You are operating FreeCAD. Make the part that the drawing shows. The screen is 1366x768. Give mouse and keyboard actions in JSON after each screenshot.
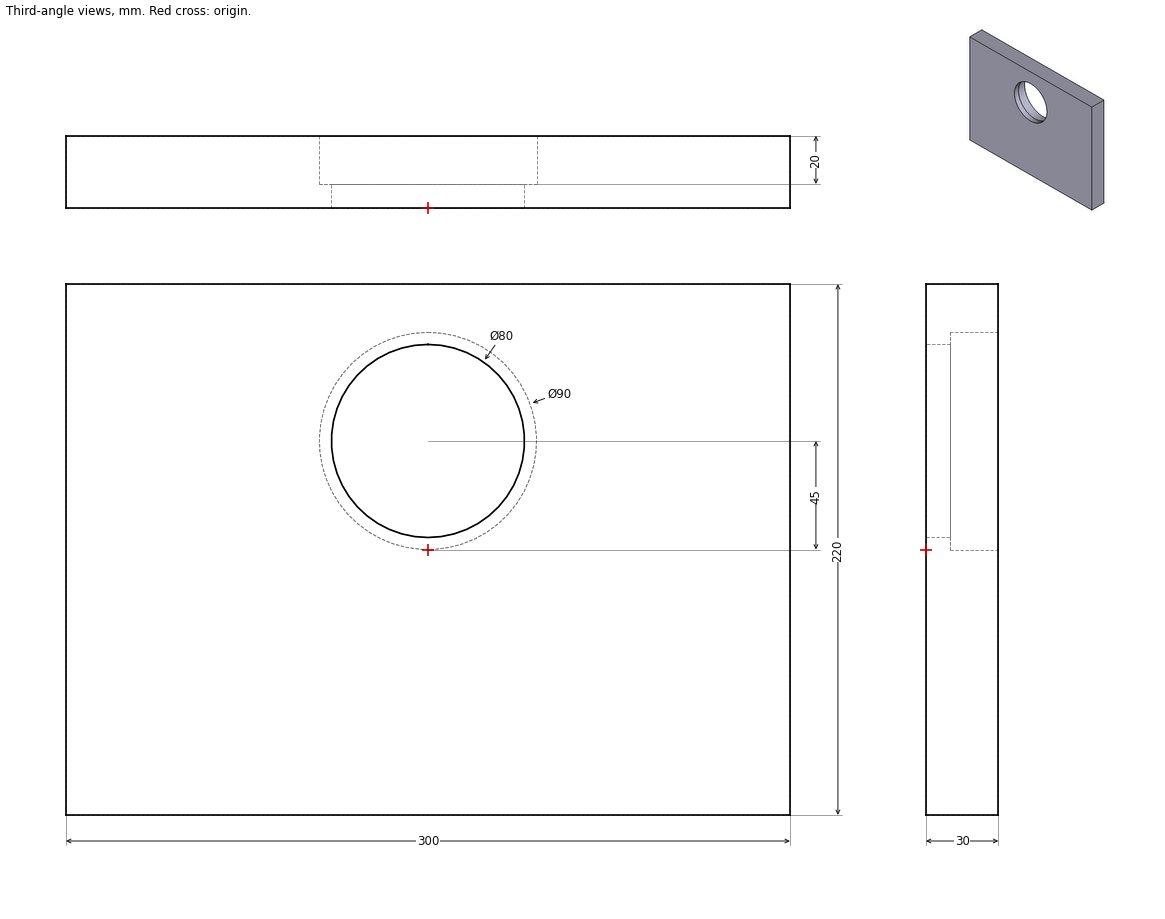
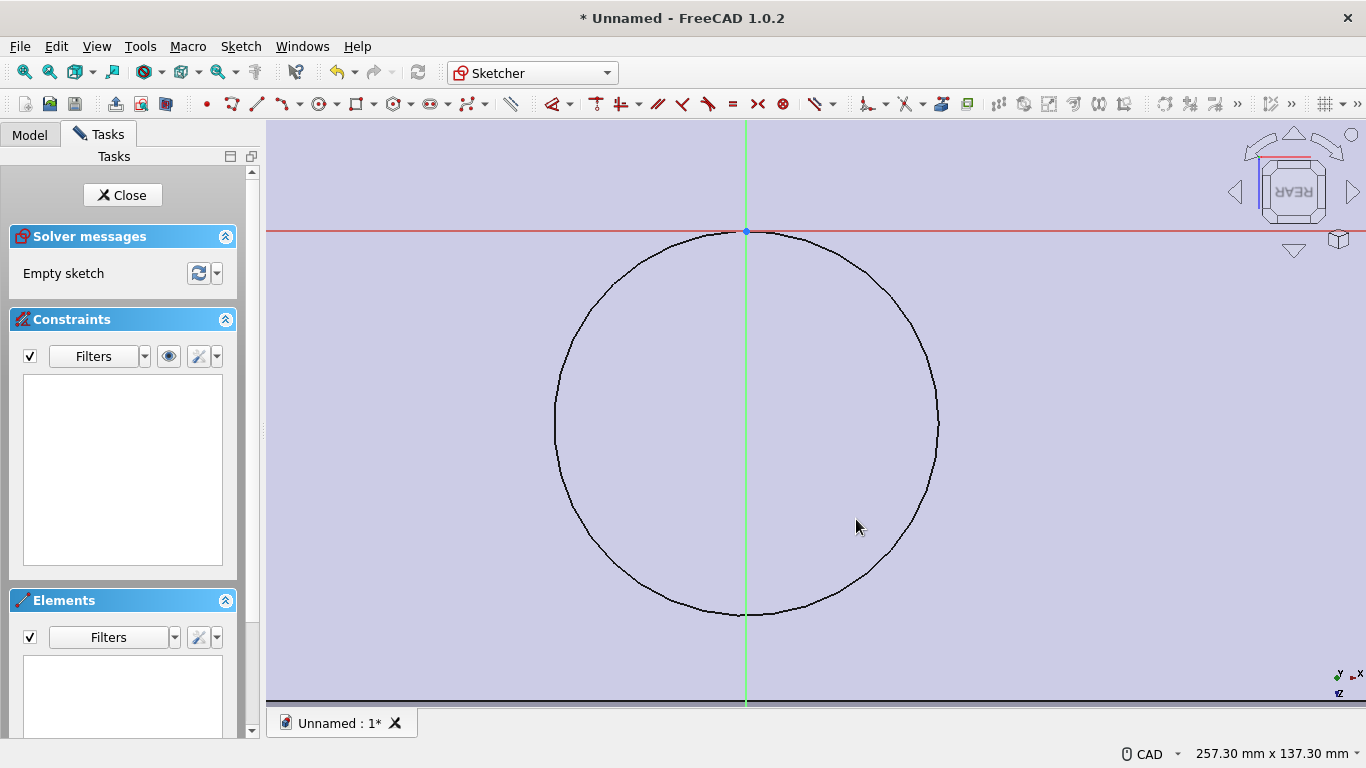
{"action": "left_click", "coordinate": [318, 104]}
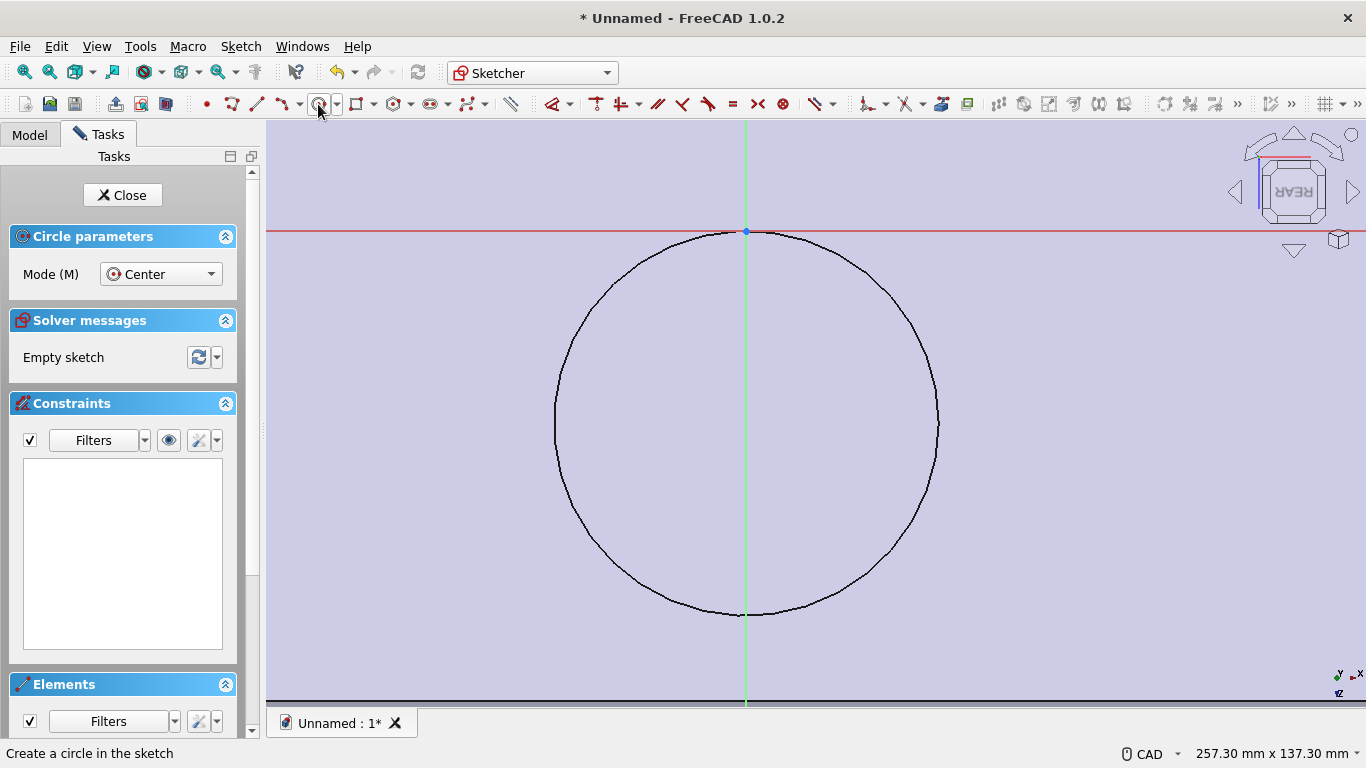
{"action": "left_click", "coordinate": [746, 423]}
{"action": "left_click", "coordinate": [867, 303]}
{"action": "key", "text": "Escape"}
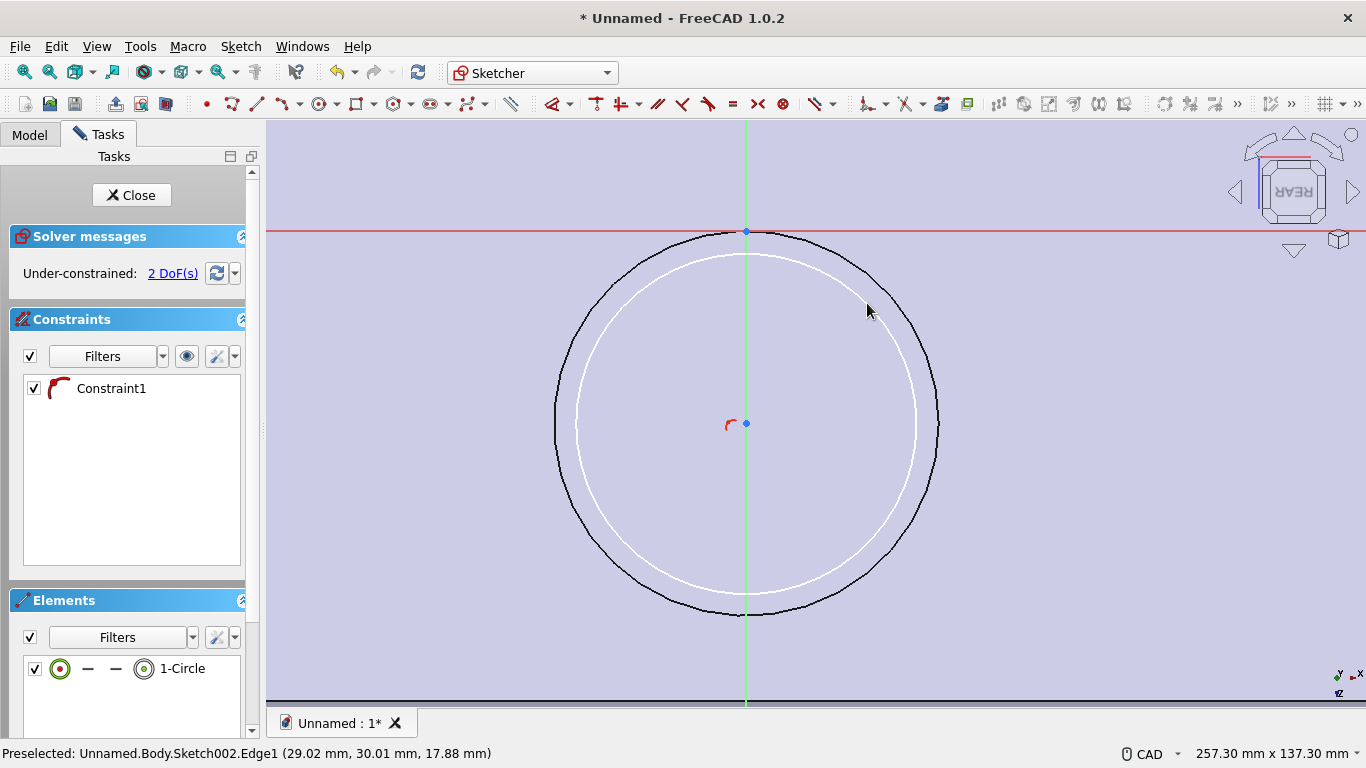
{"action": "left_click", "coordinate": [552, 104]}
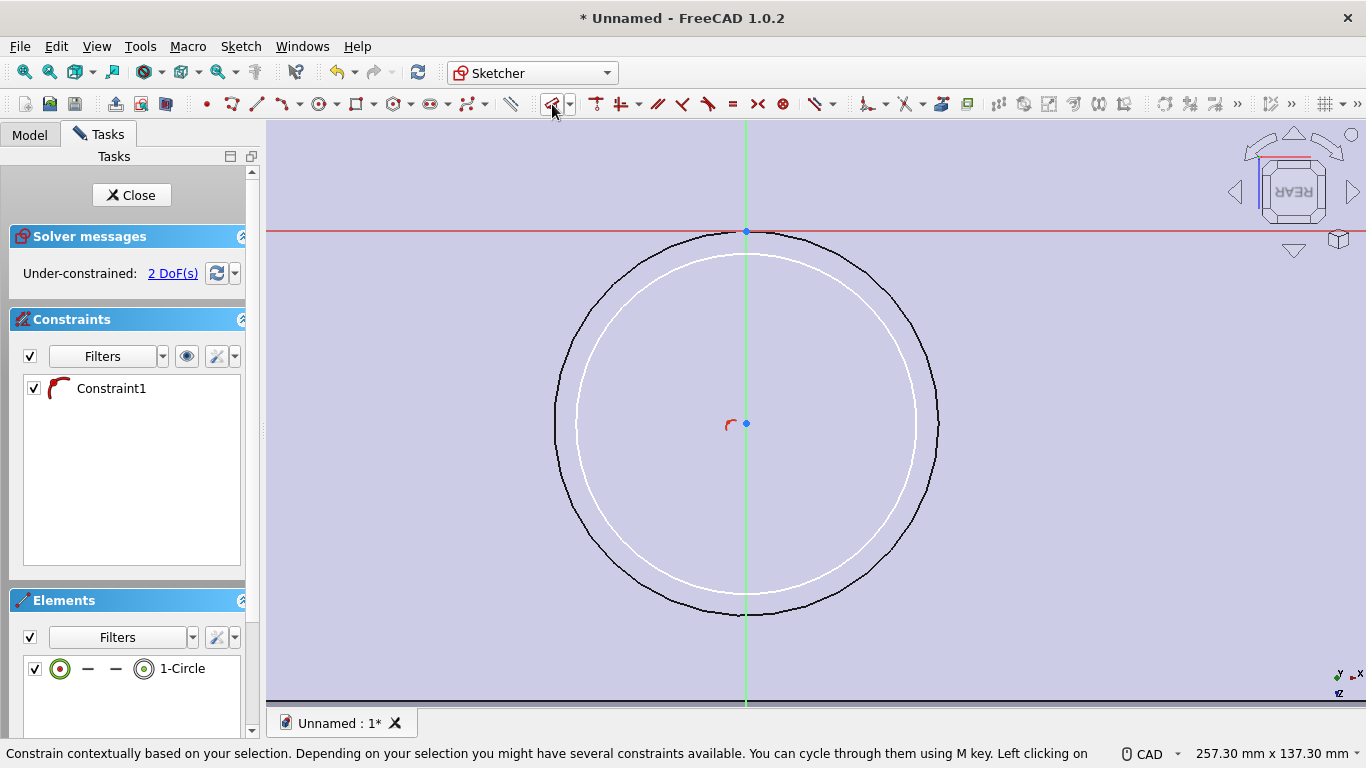
{"action": "left_click", "coordinate": [866, 303]}
{"action": "left_click", "coordinate": [889, 280]}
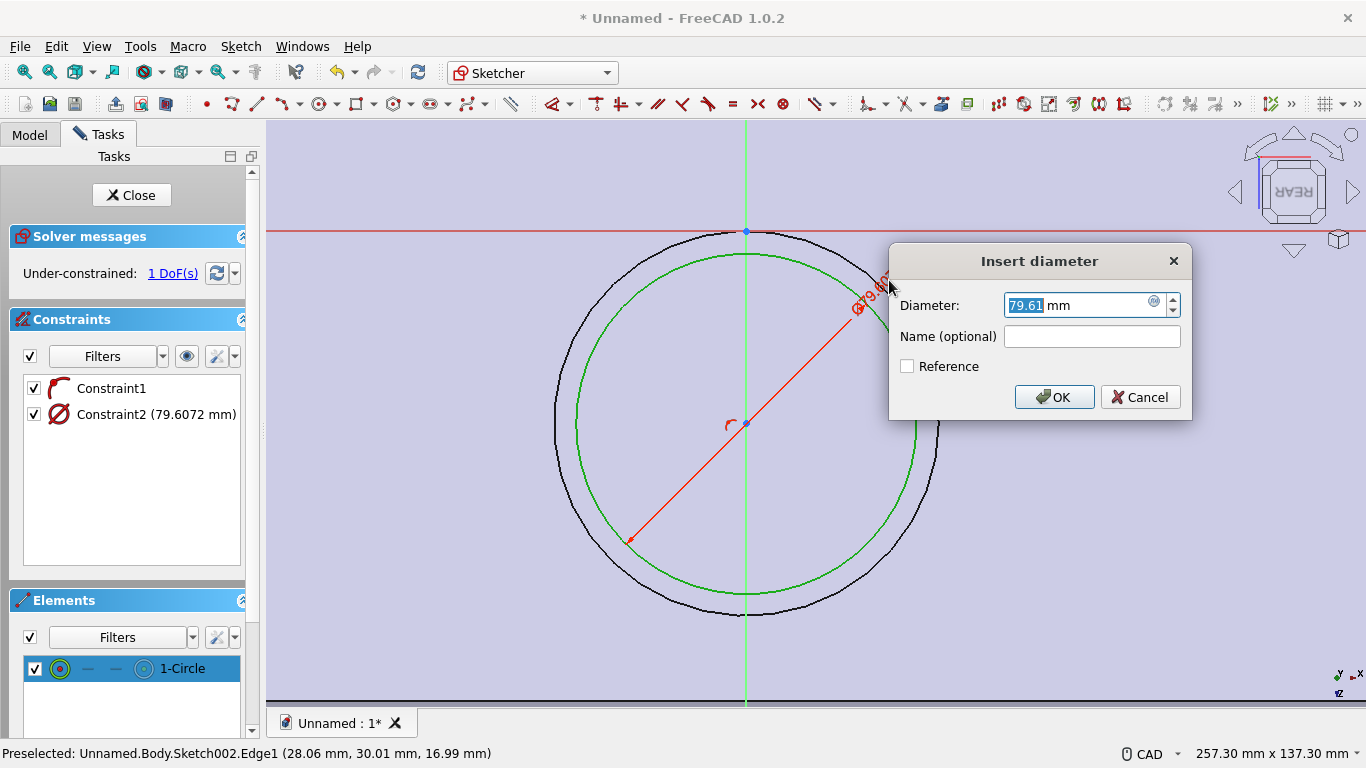
{"action": "type", "text": "80"}
{"action": "key", "text": "Return"}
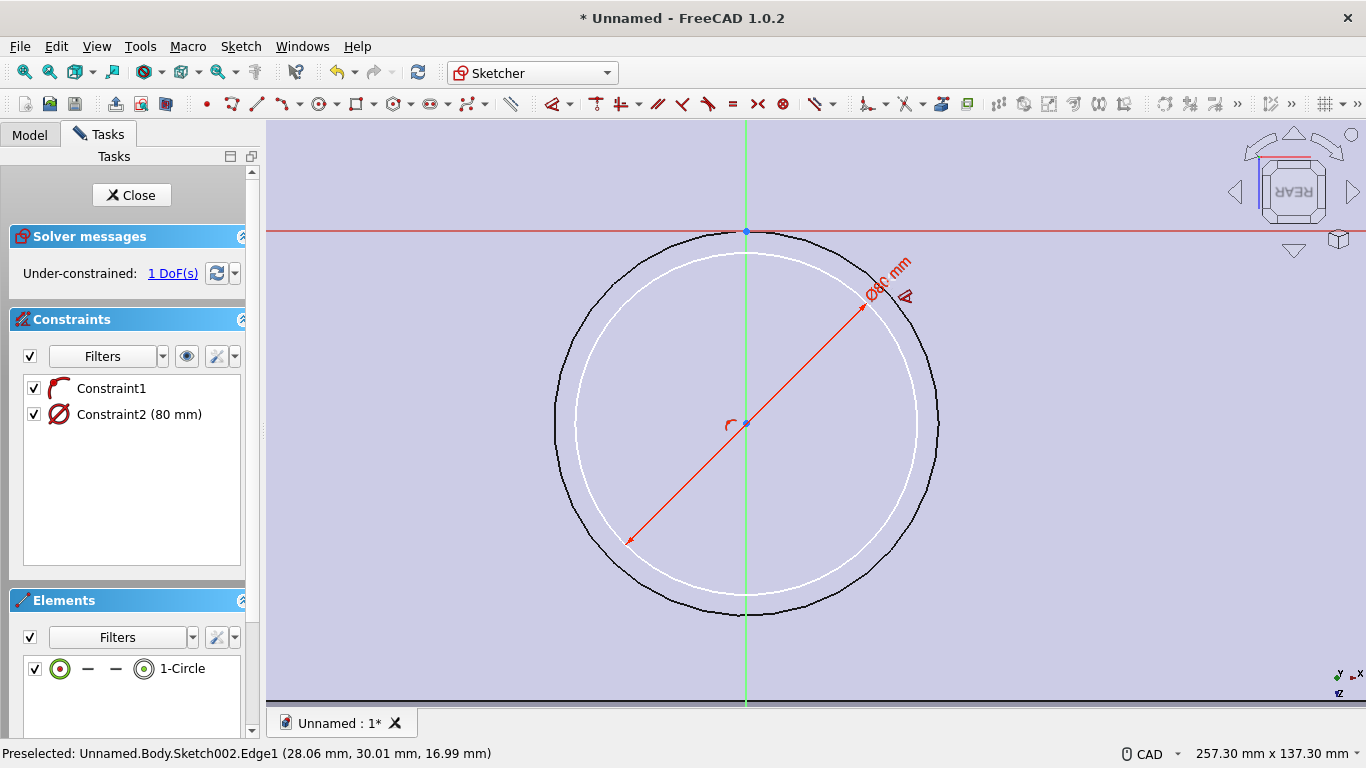
{"action": "left_click", "coordinate": [746, 424]}
{"action": "left_click", "coordinate": [780, 328]}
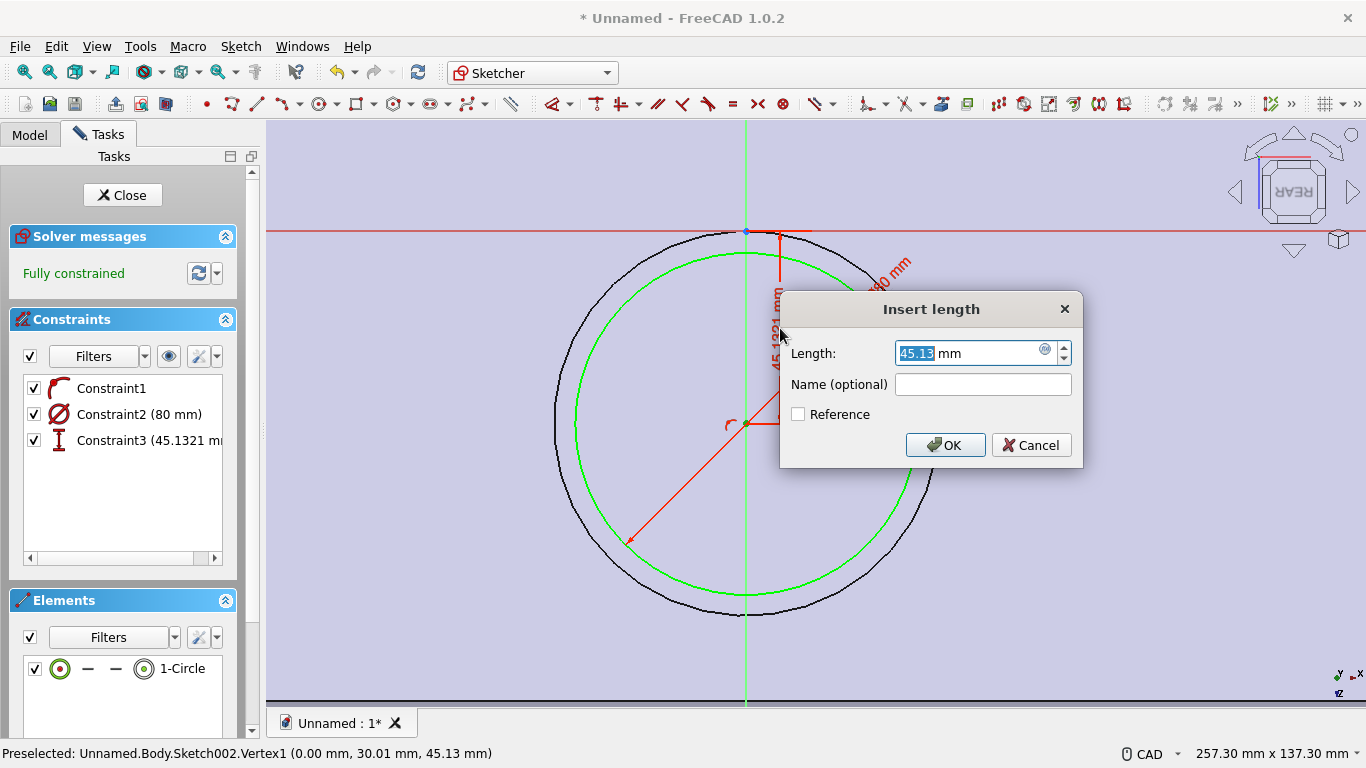
{"action": "type", "text": "45"}
{"action": "key", "text": "Return"}
{"action": "key", "text": "Escape"}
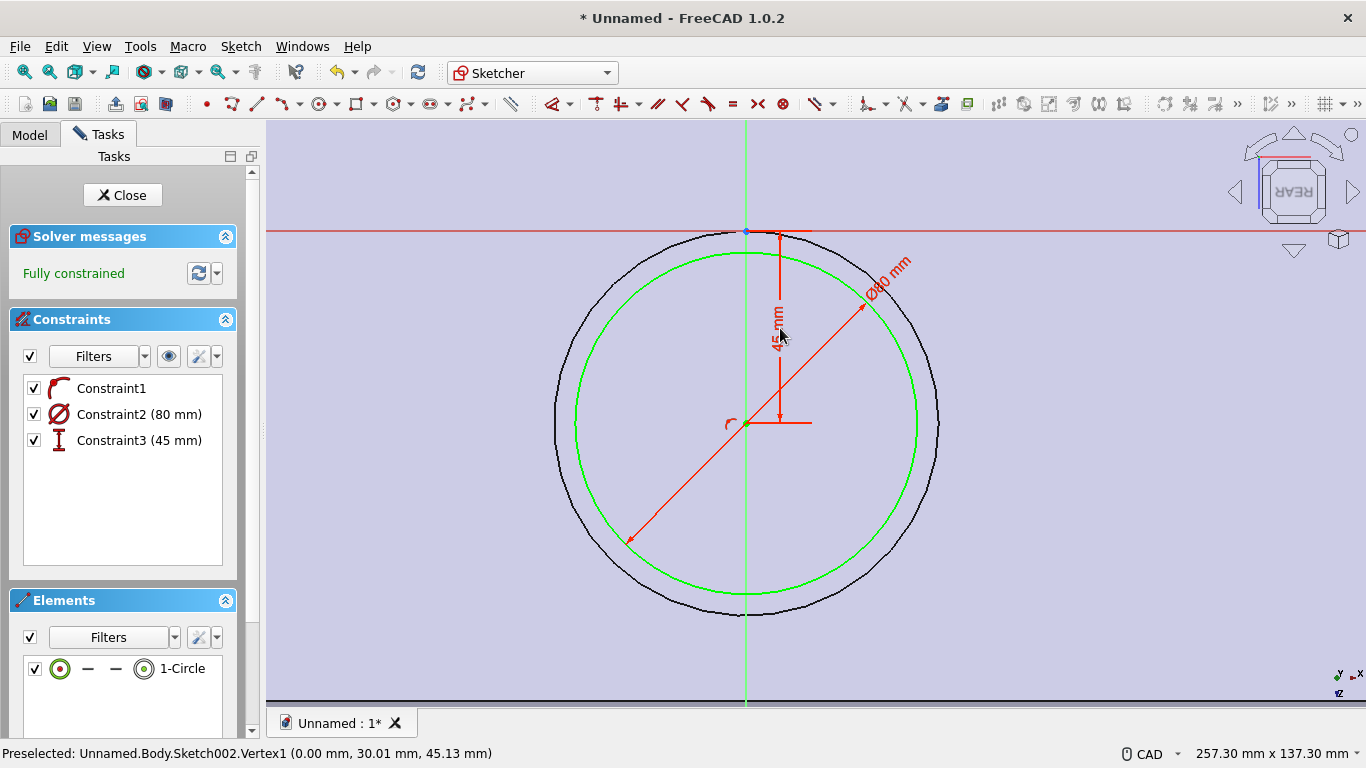
{"action": "left_click", "coordinate": [123, 195]}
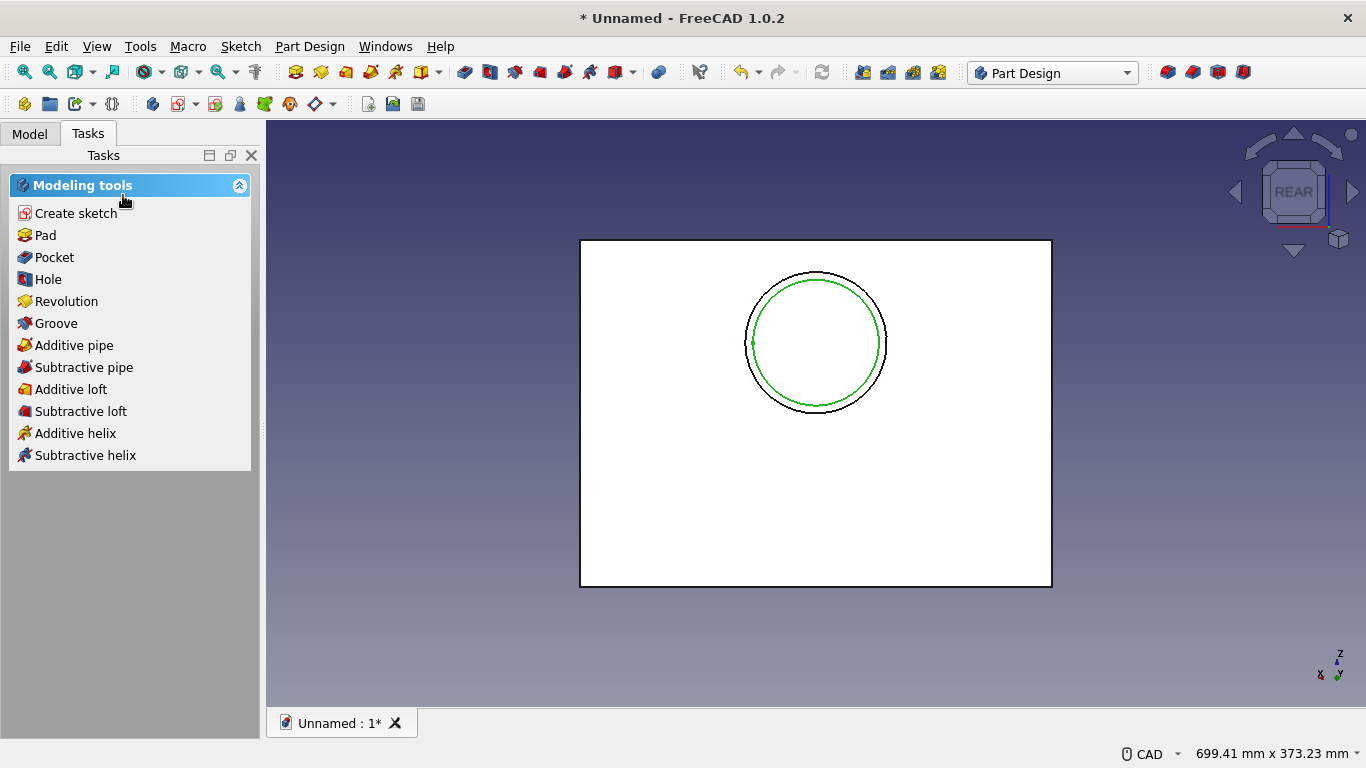
{"action": "left_click", "coordinate": [465, 72]}